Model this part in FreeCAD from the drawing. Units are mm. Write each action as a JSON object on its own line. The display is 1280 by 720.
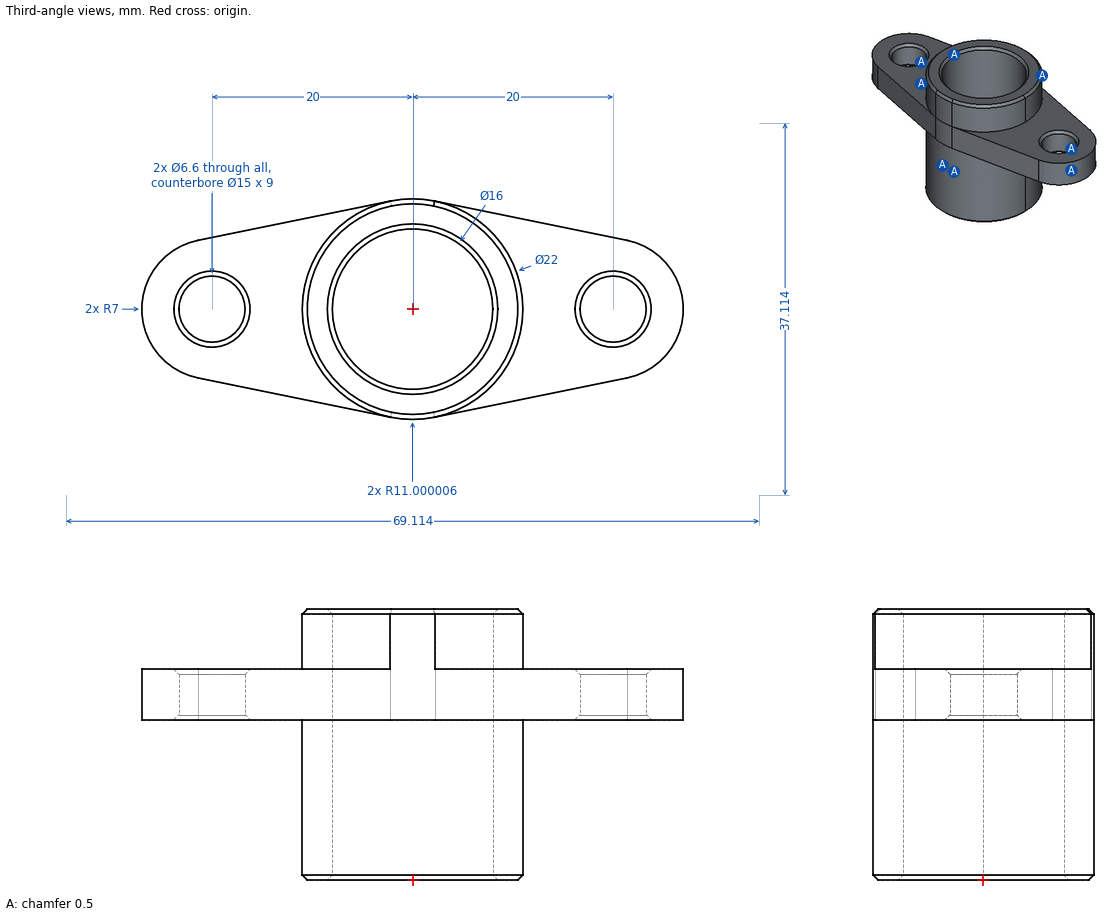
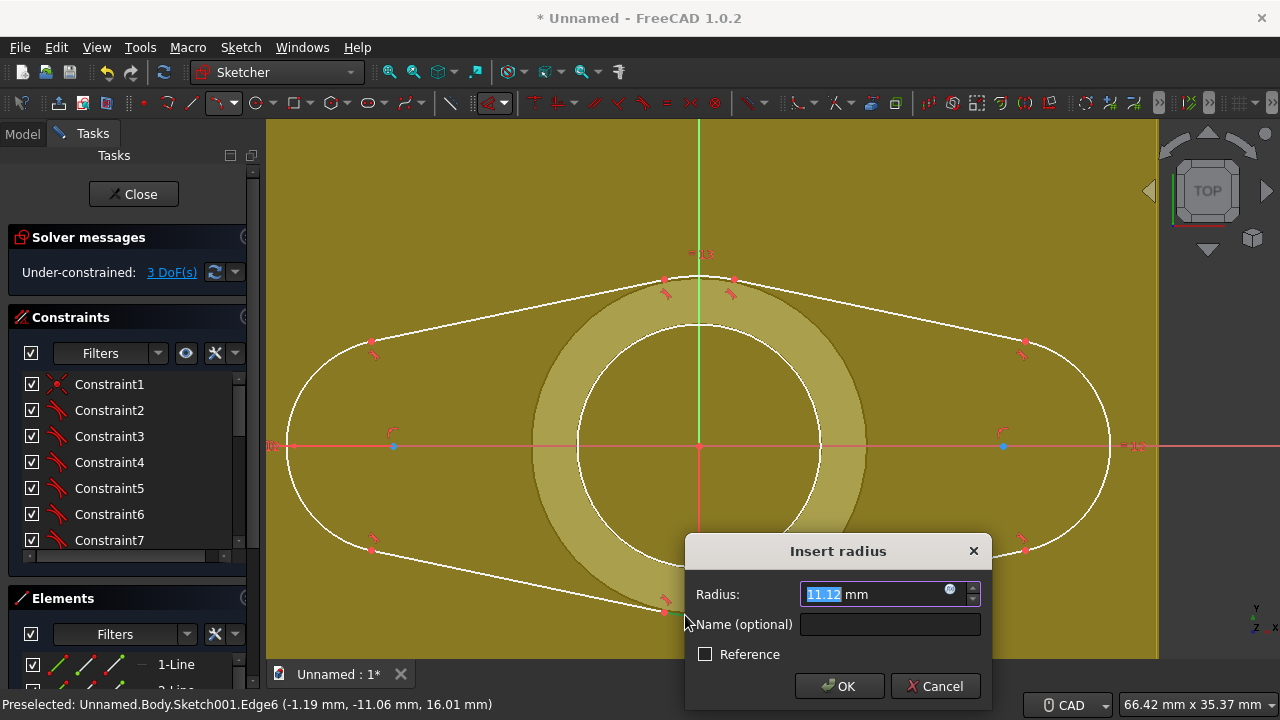
{"action": "type", "text": "11.000006"}
{"action": "key", "text": "Return"}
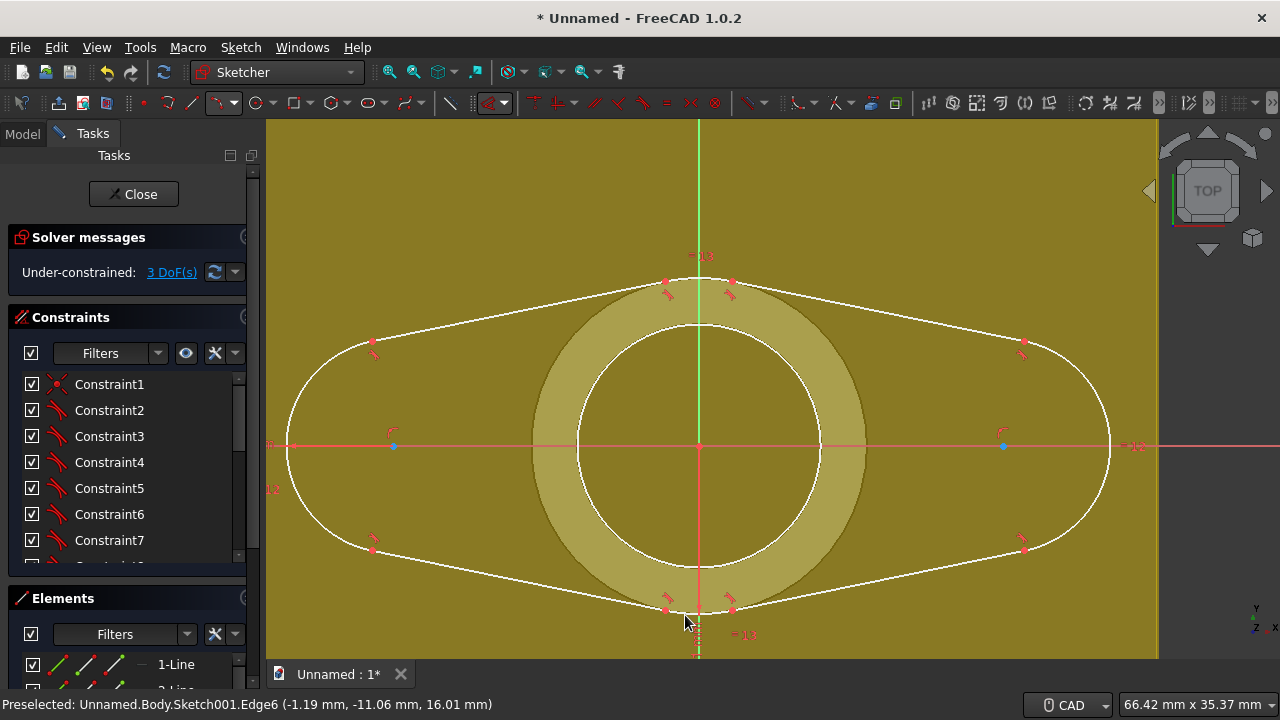
{"action": "left_click", "coordinate": [785, 360]}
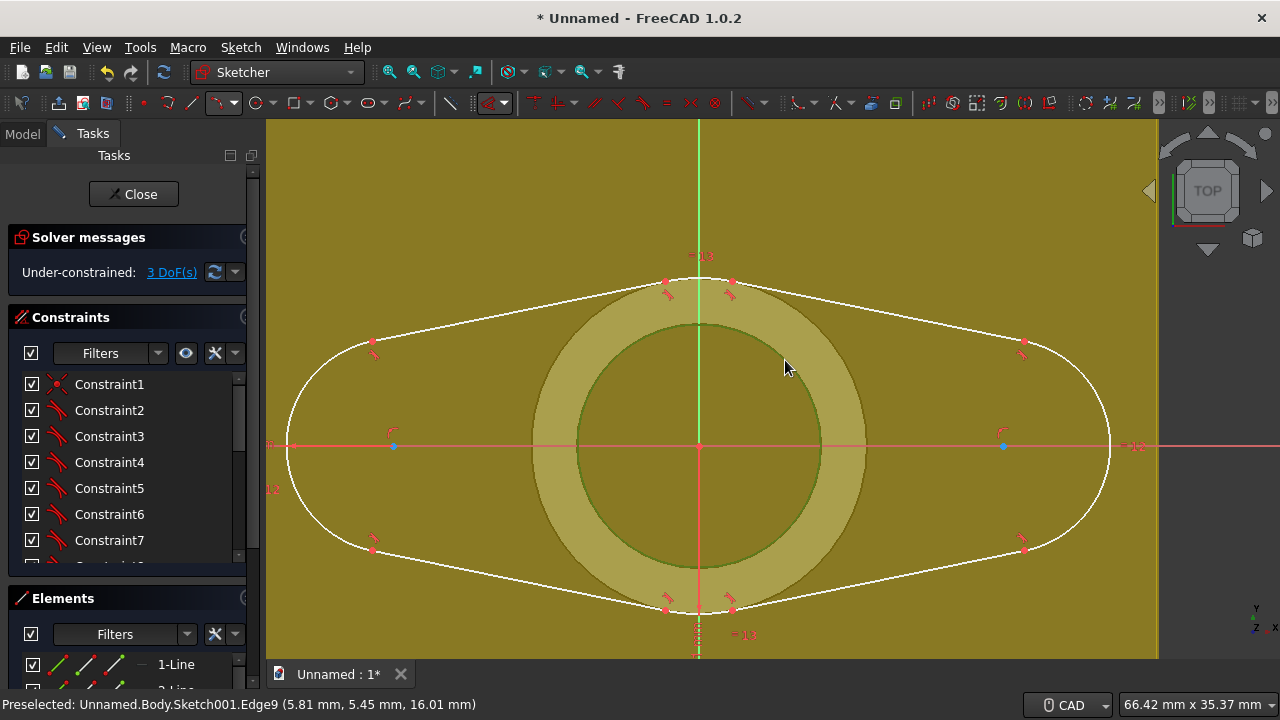
{"action": "key", "text": "k o"}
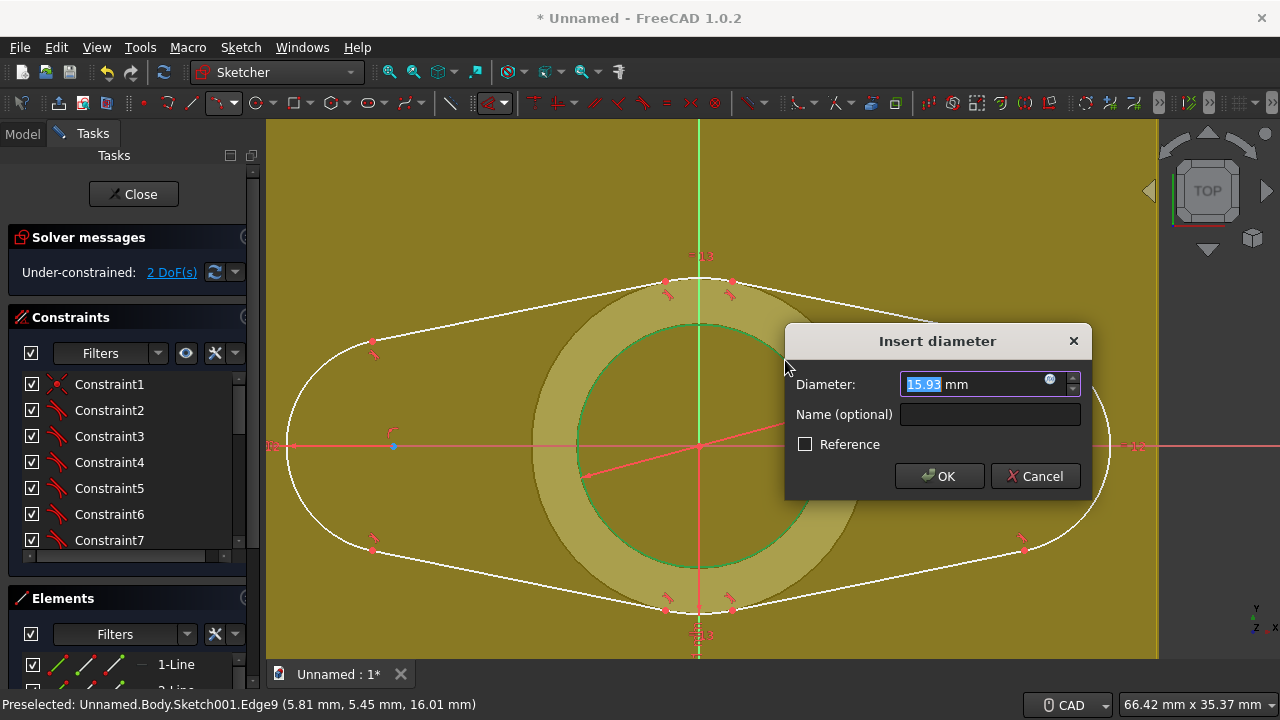
{"action": "type", "text": "16"}
{"action": "key", "text": "Return"}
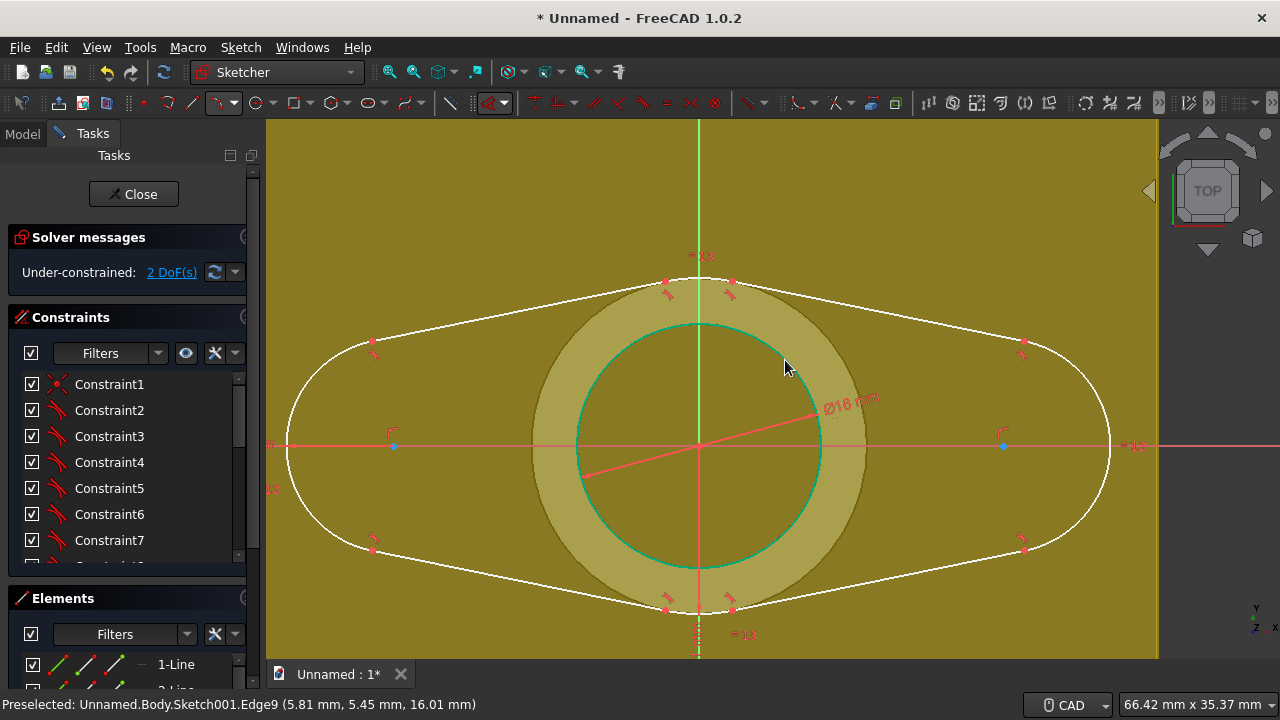
{"action": "left_click", "coordinate": [393, 446]}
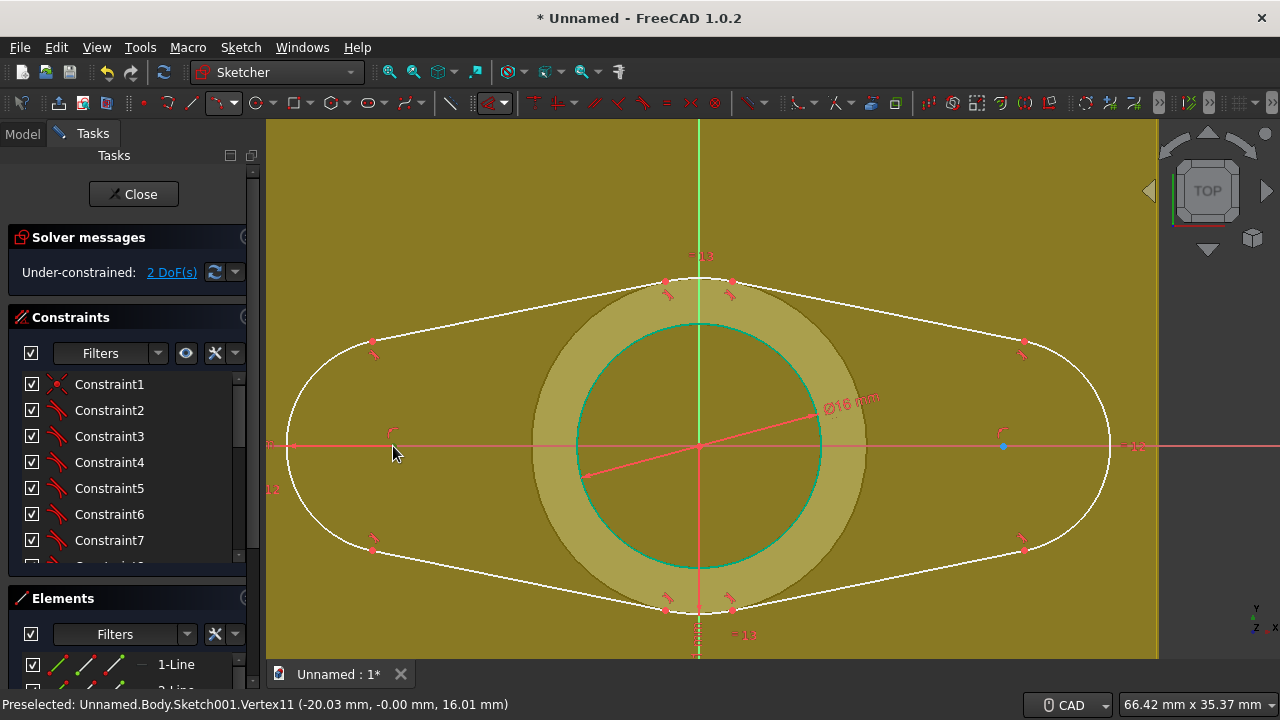
{"action": "key", "text": "l"}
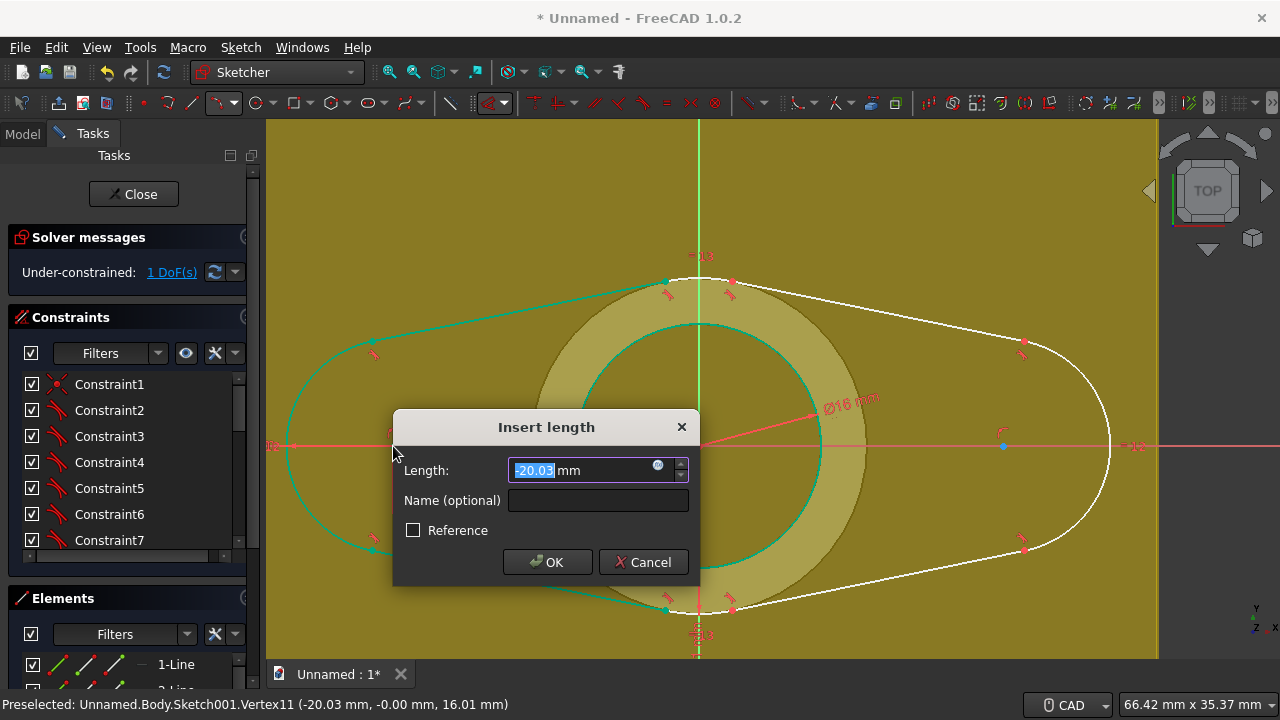
{"action": "type", "text": "-20"}
{"action": "key", "text": "Return"}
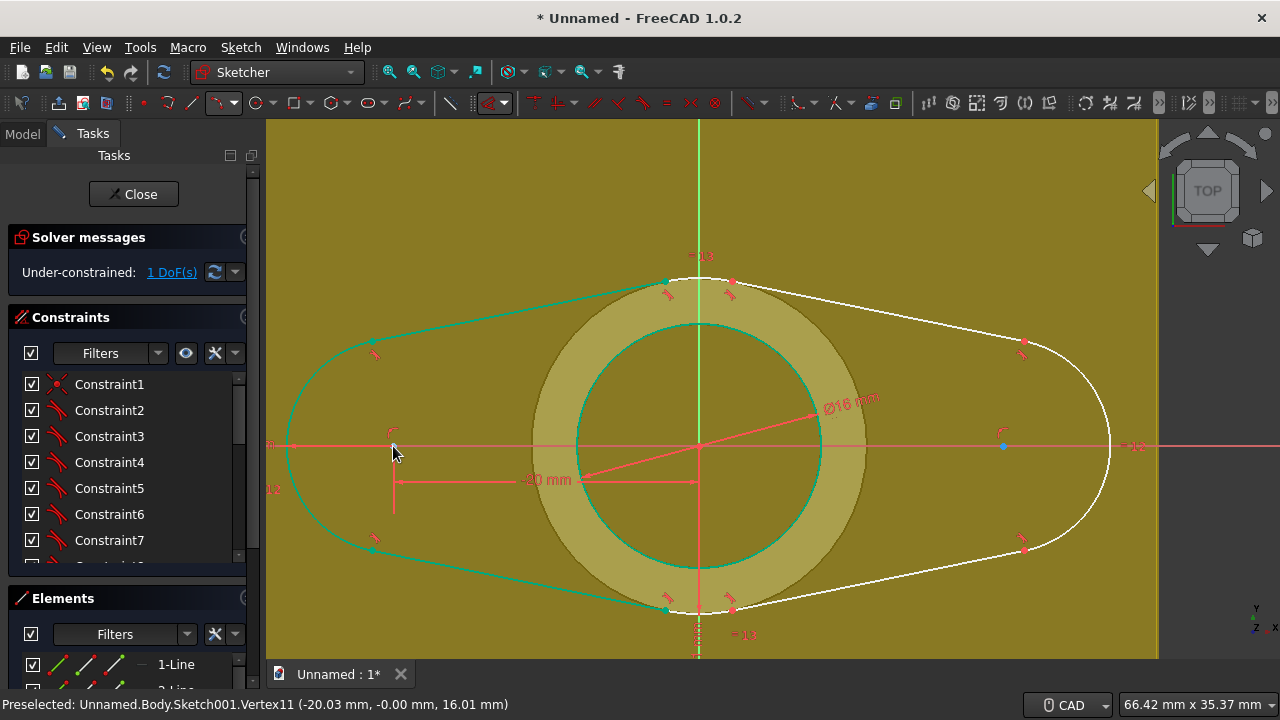
{"action": "left_click", "coordinate": [1003, 446]}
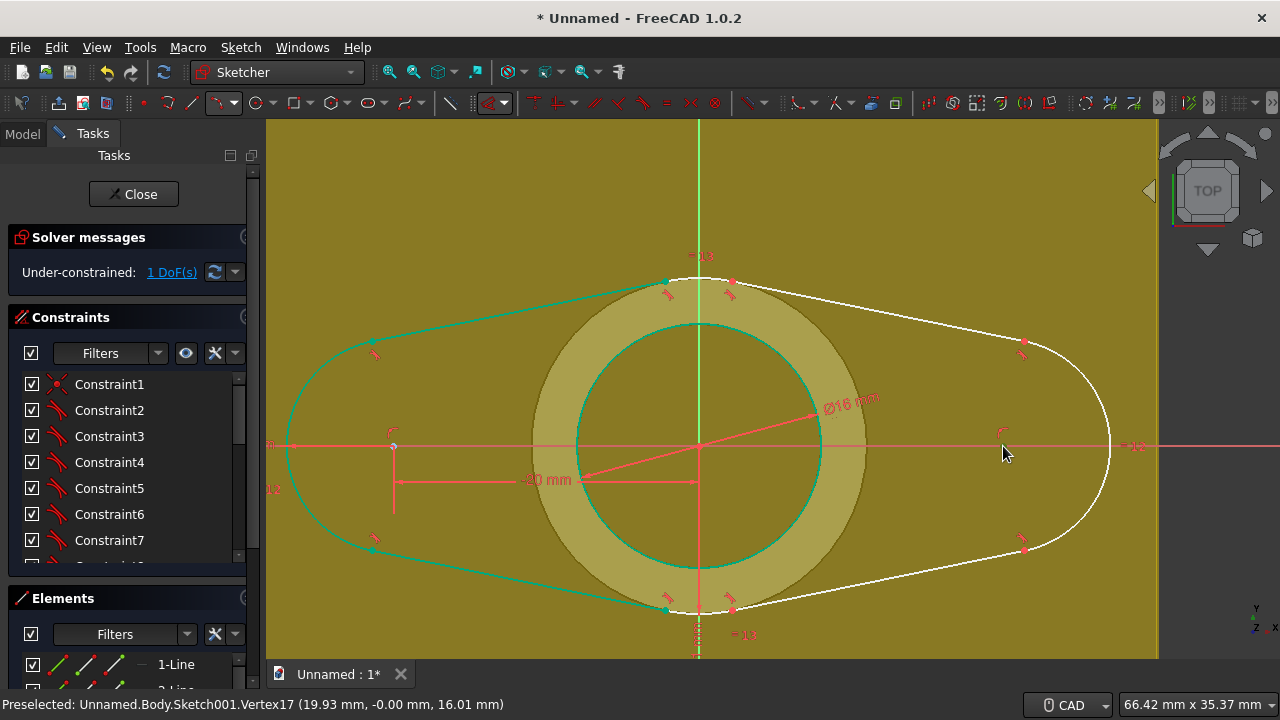
{"action": "key", "text": "l"}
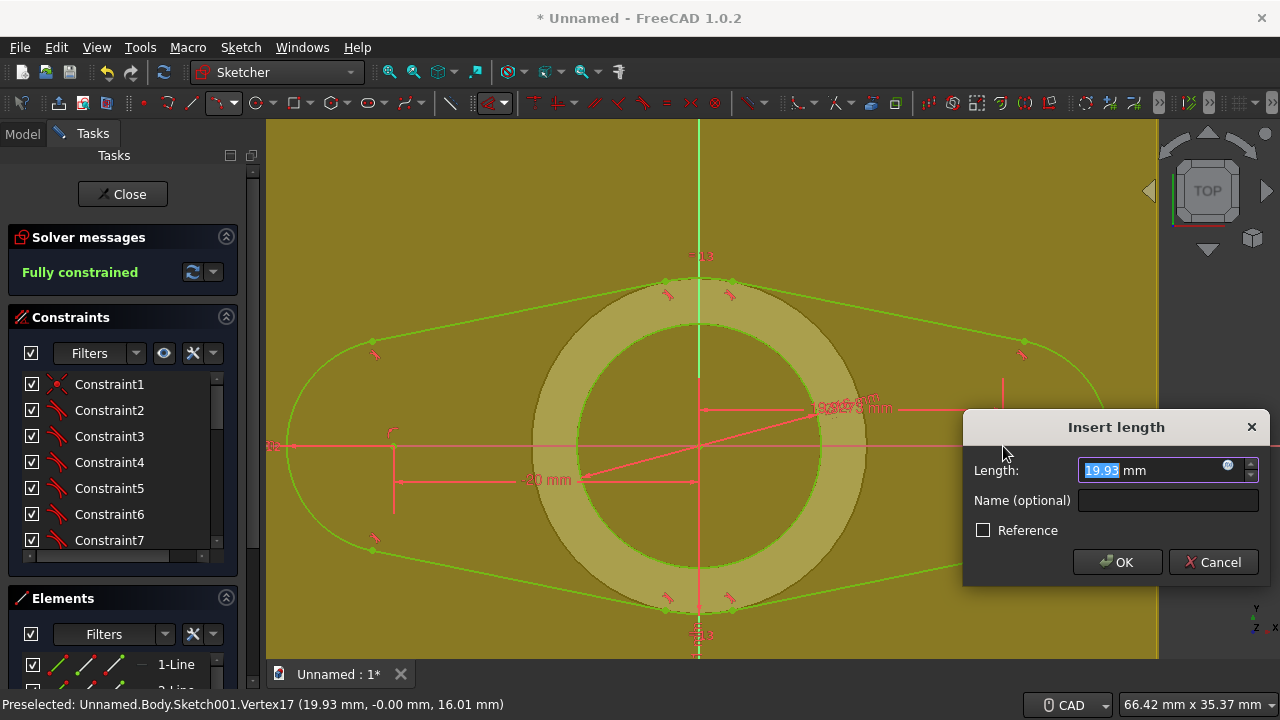
{"action": "type", "text": "20"}
{"action": "key", "text": "Return"}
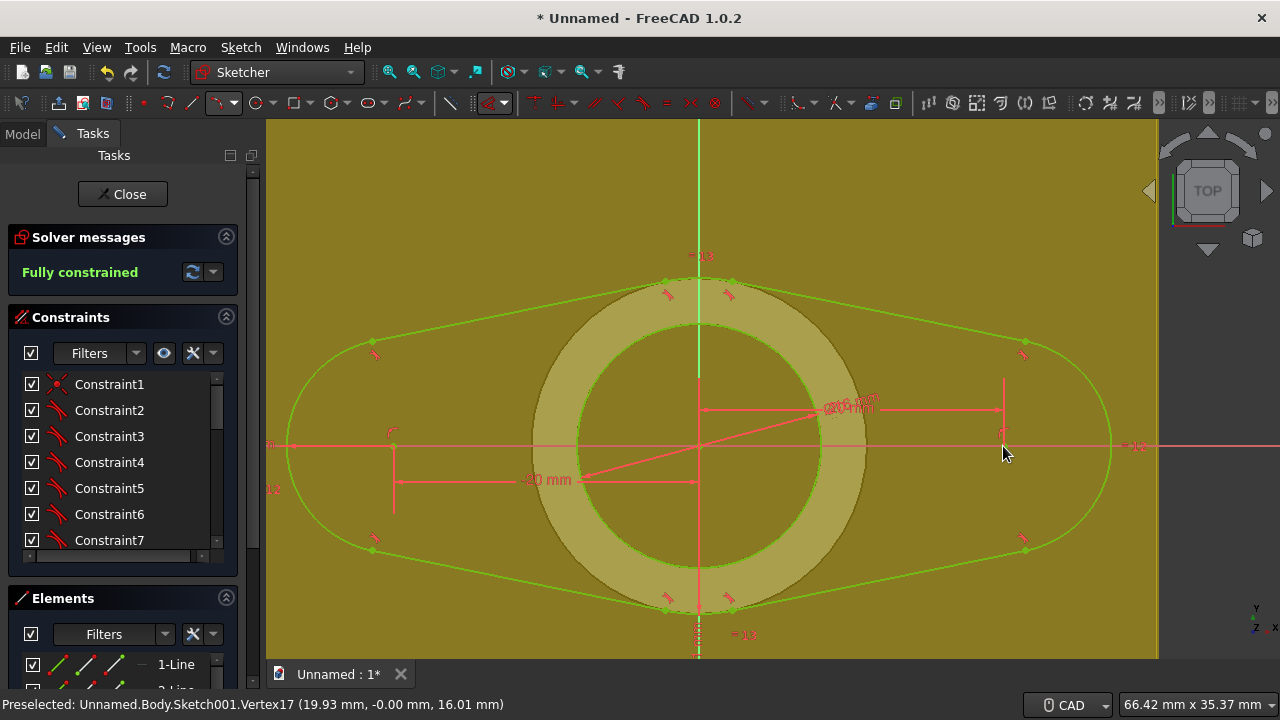
{"action": "left_click", "coordinate": [123, 194]}